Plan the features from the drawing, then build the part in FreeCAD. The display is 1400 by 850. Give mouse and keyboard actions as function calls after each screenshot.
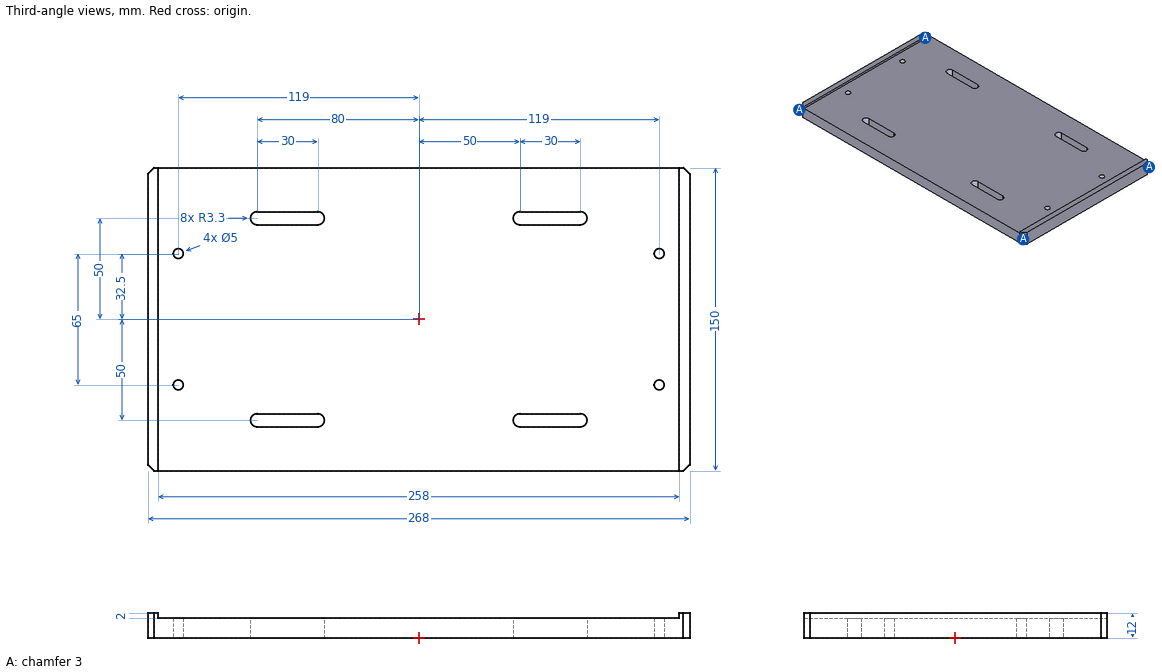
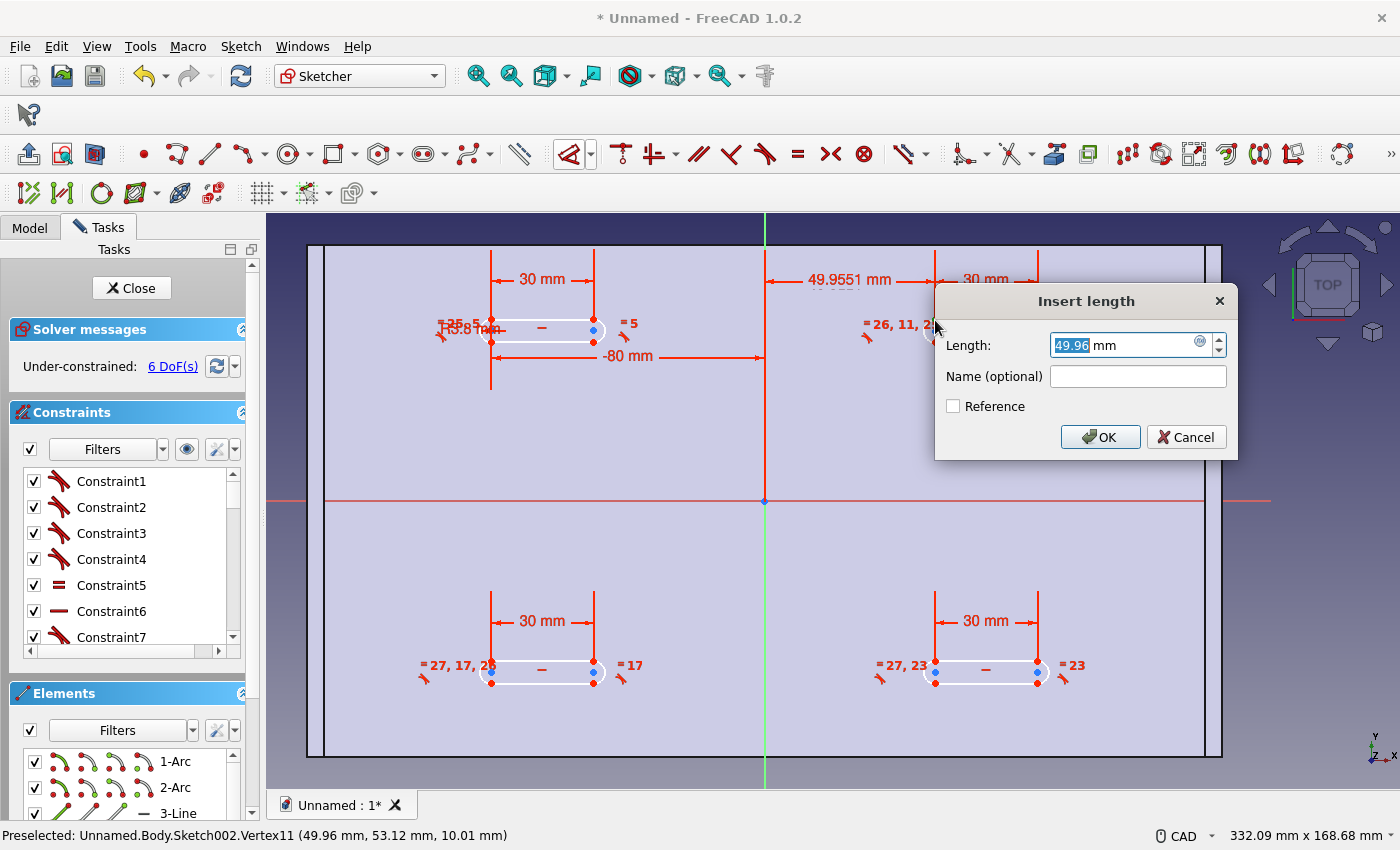
text(50)
key(Return)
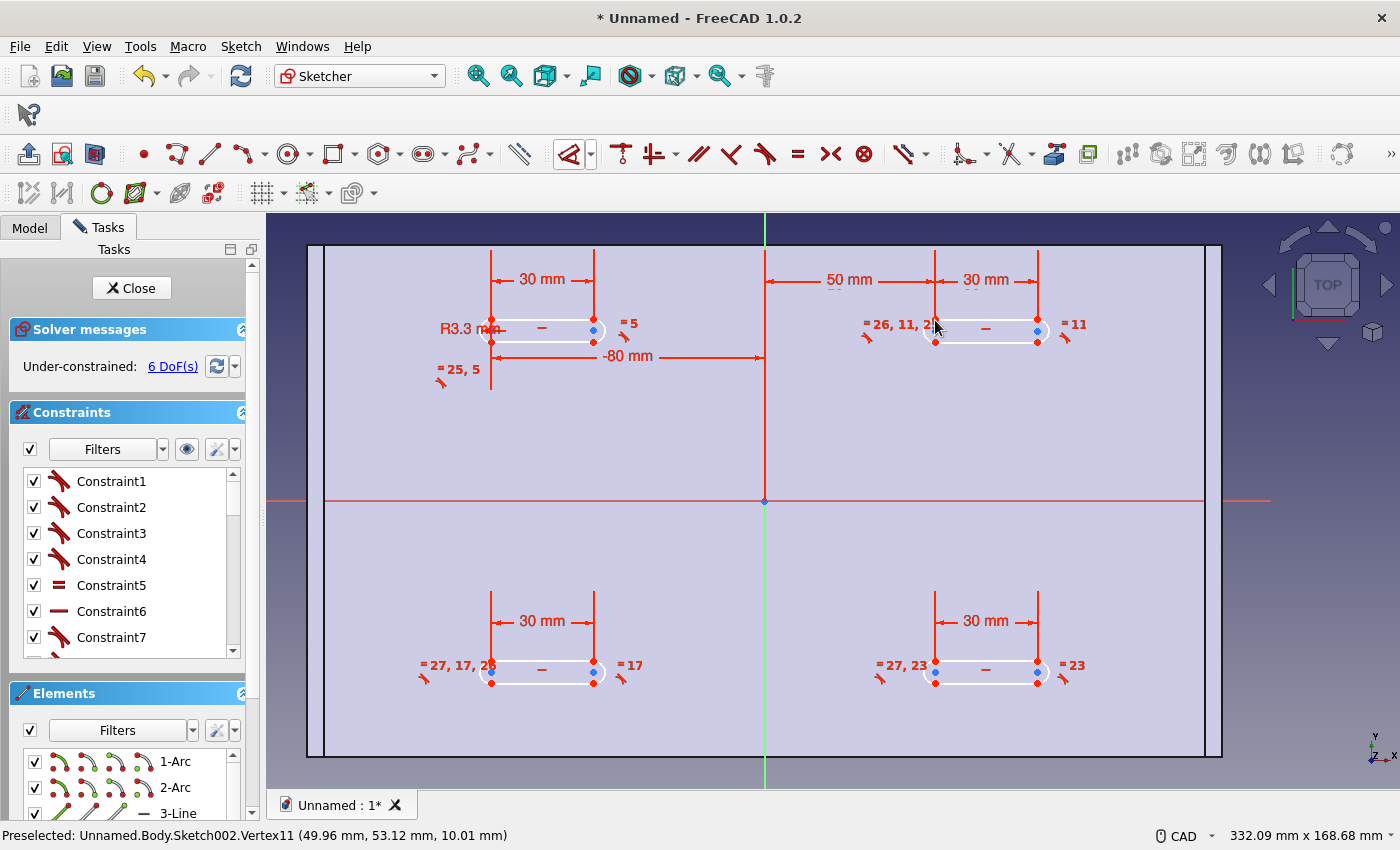
click(491, 661)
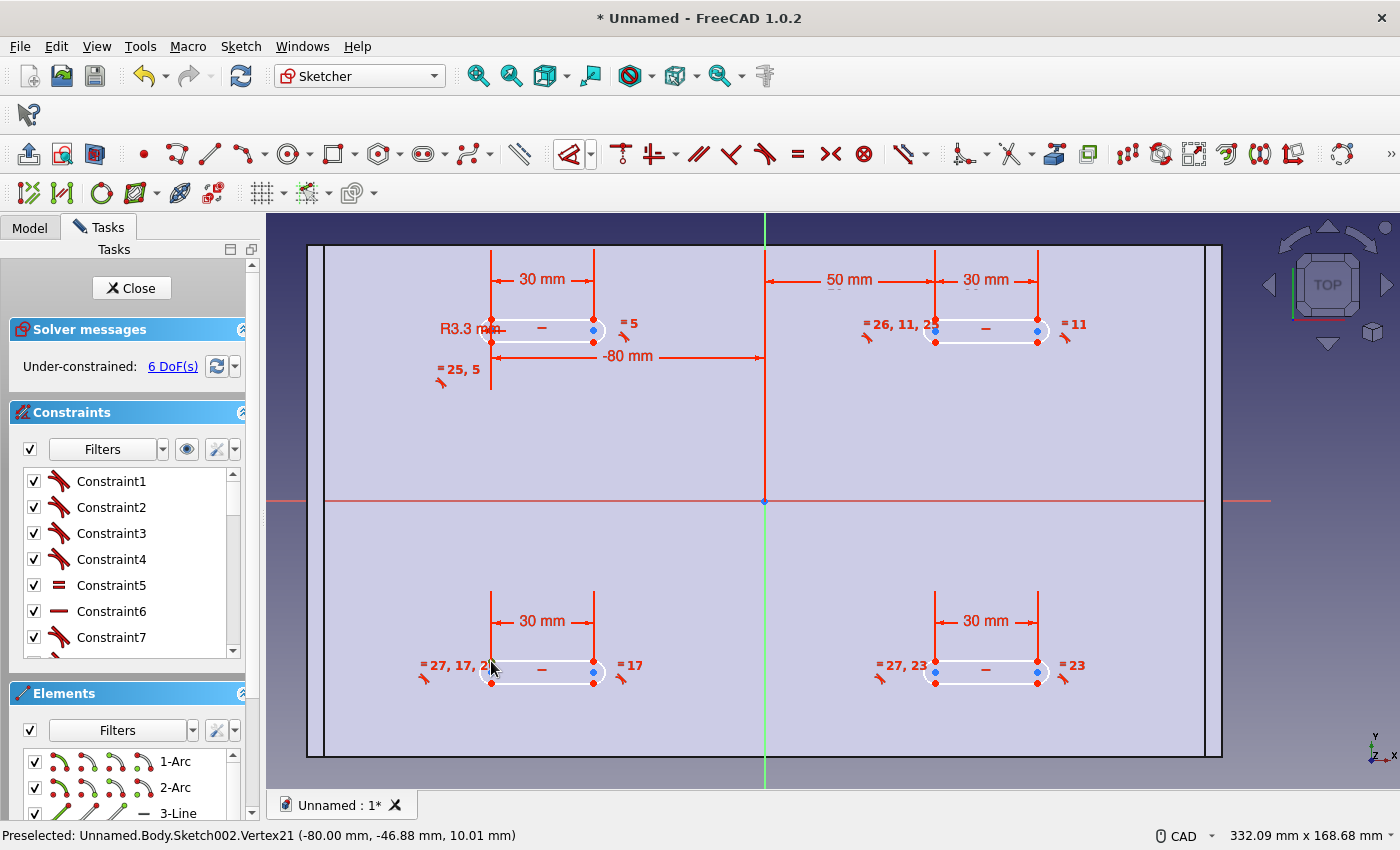
click(590, 154)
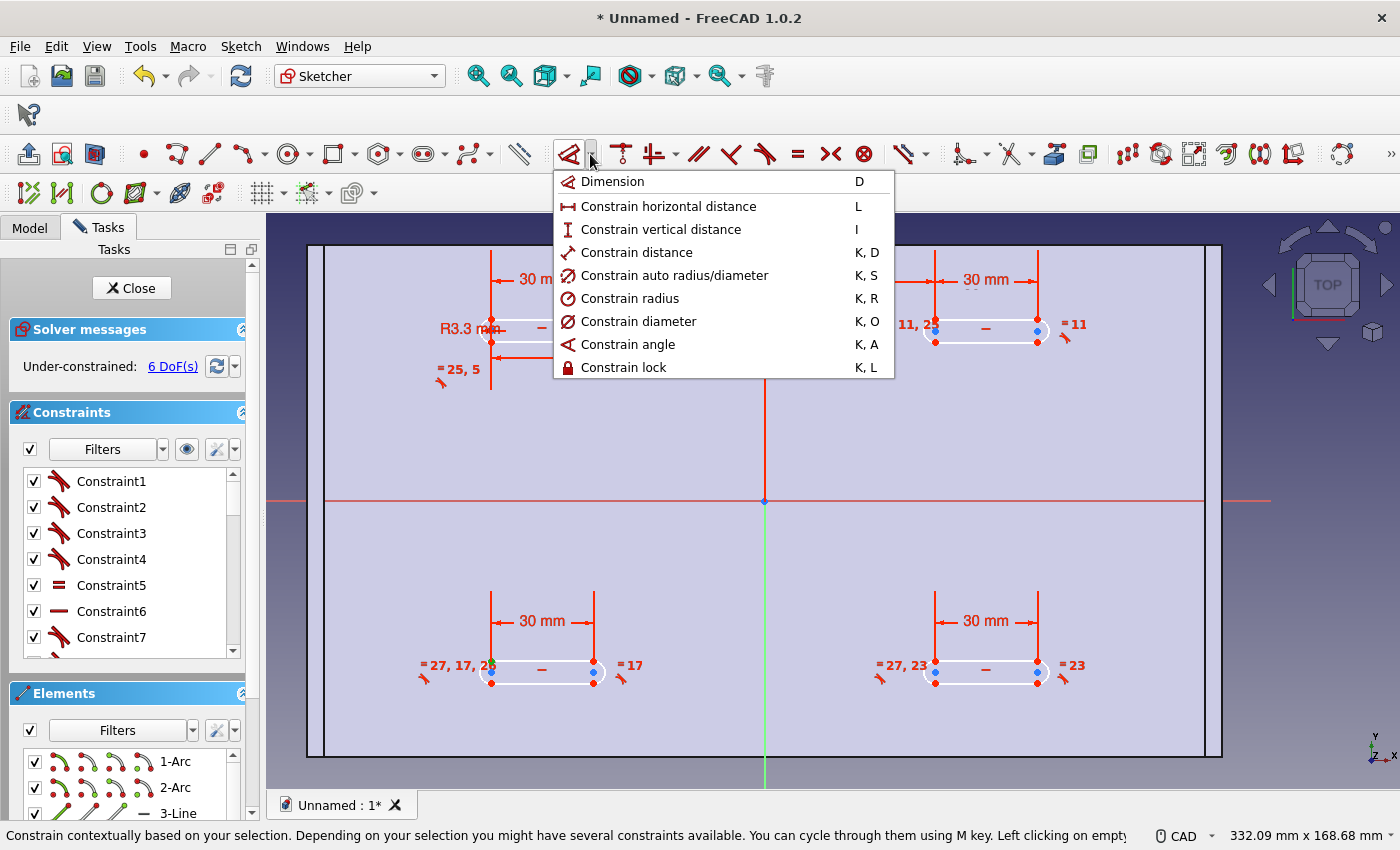
click(724, 206)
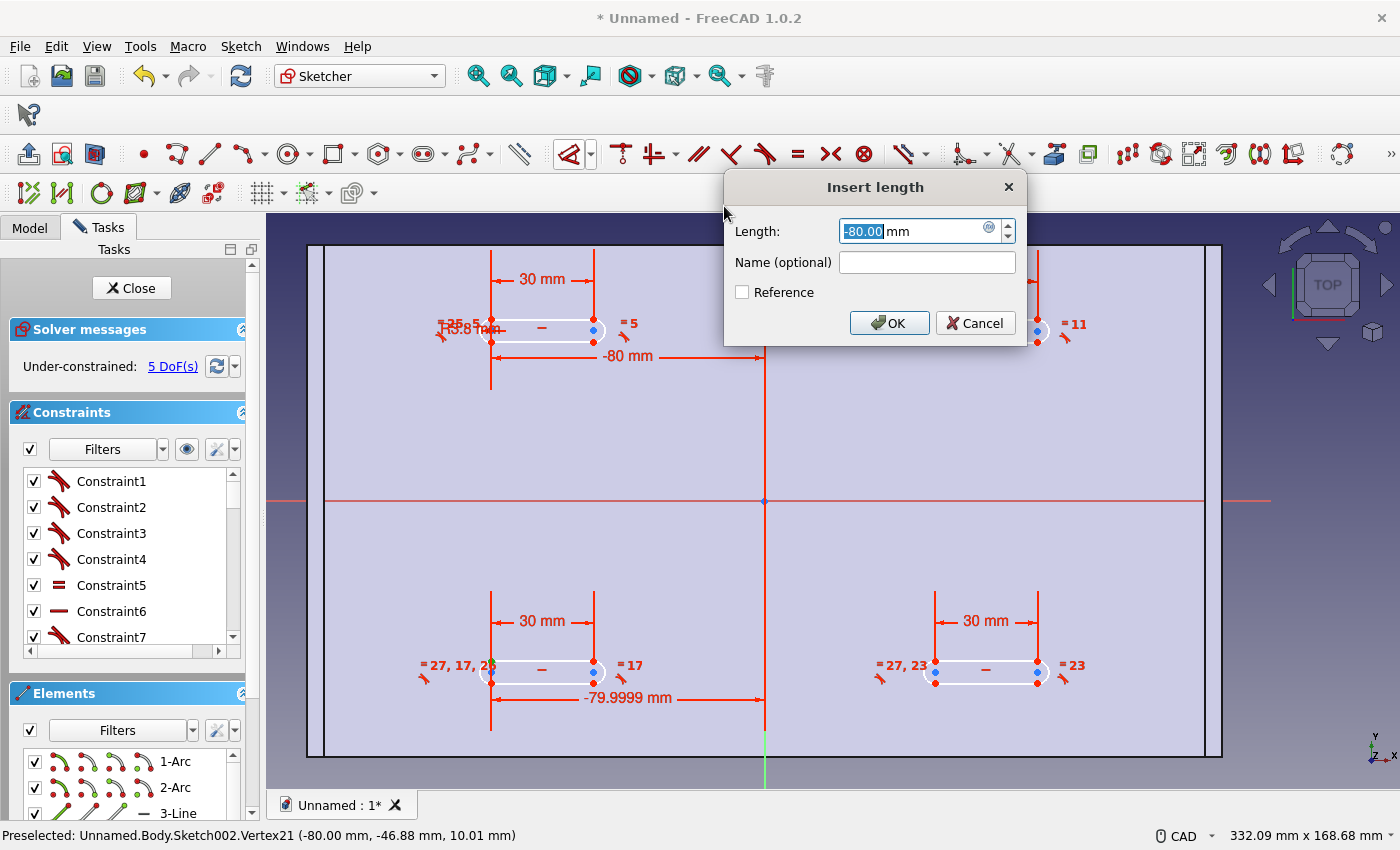
text(-80)
key(Return)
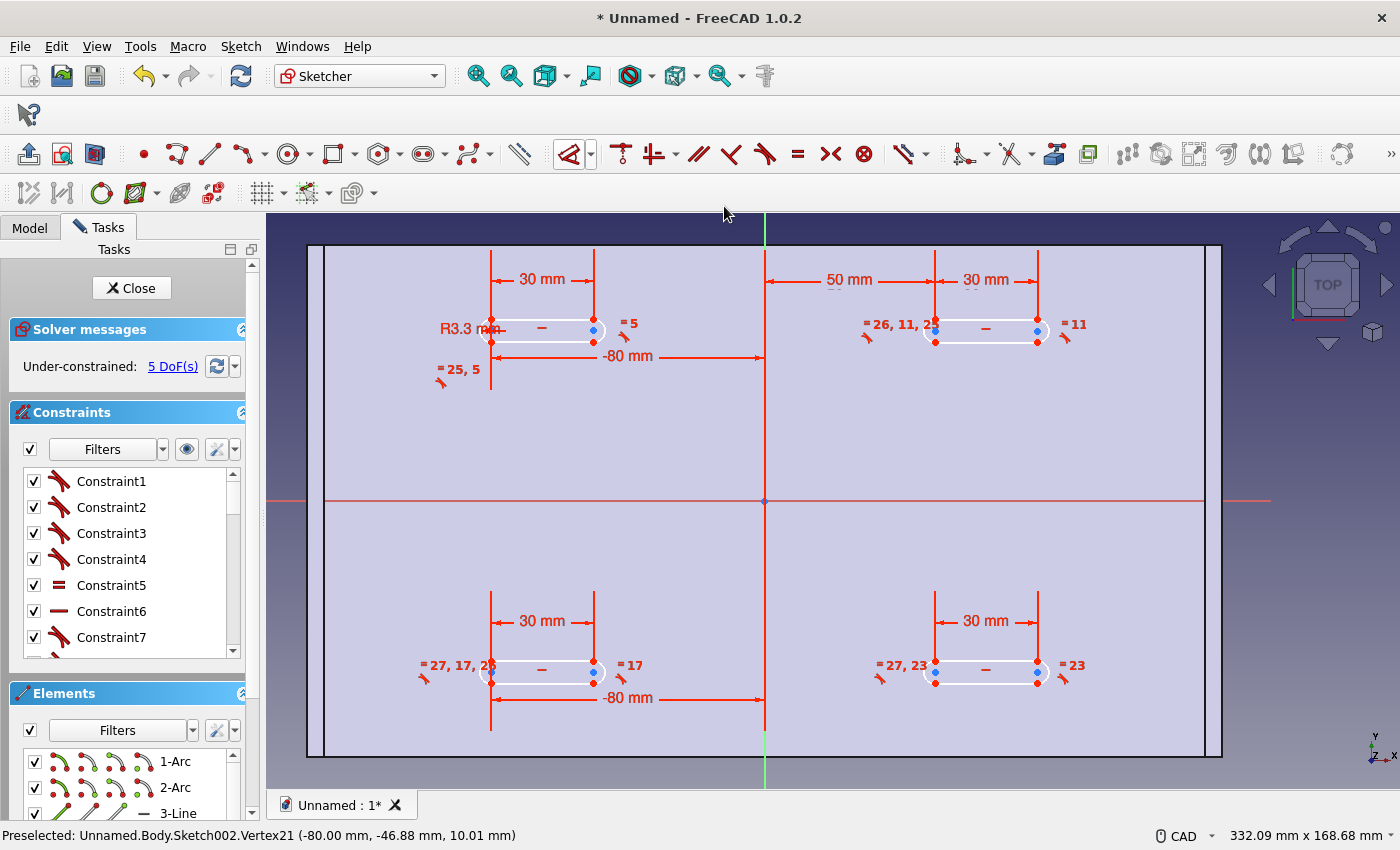
click(935, 661)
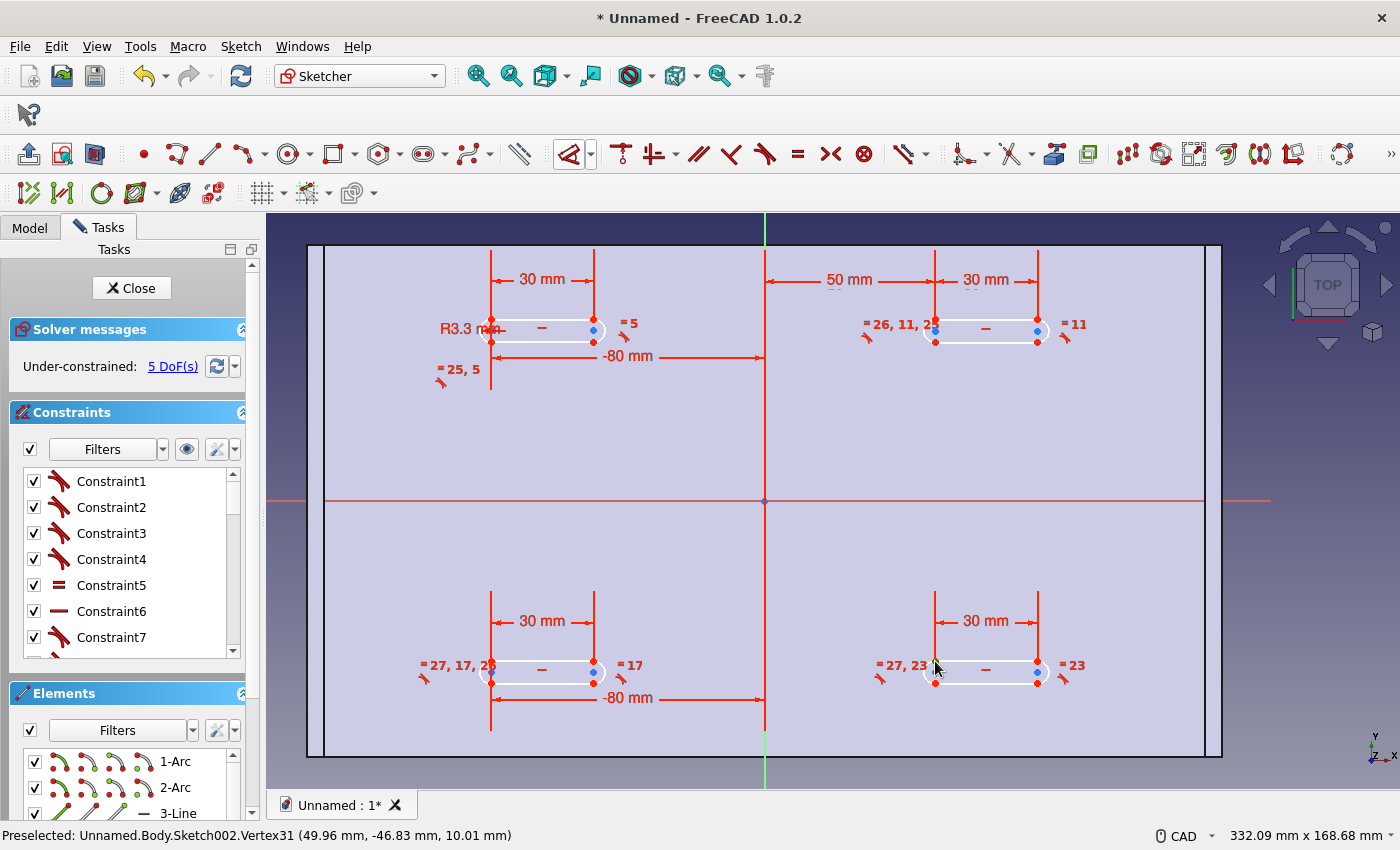
key(l)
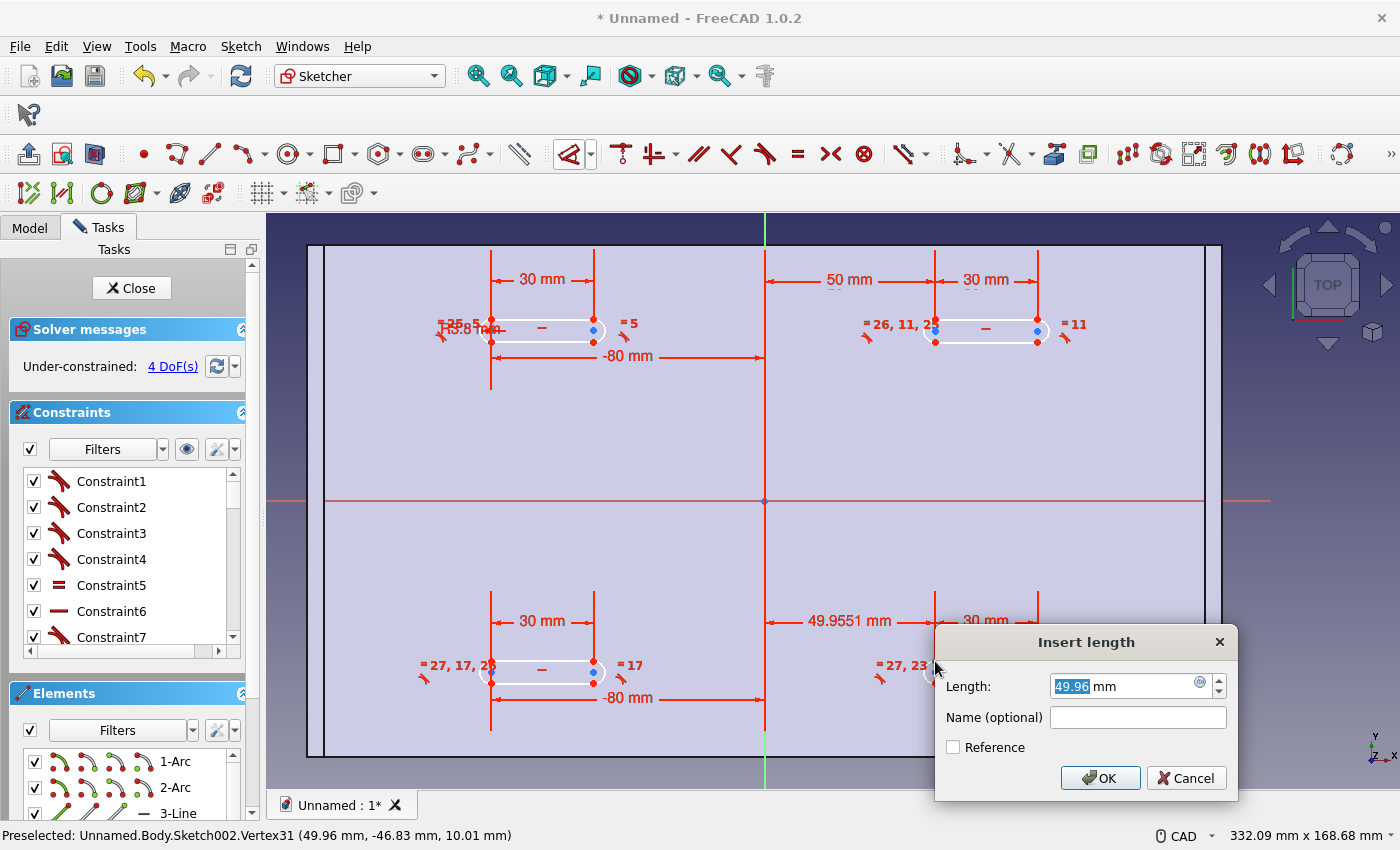
text(50)
key(Return)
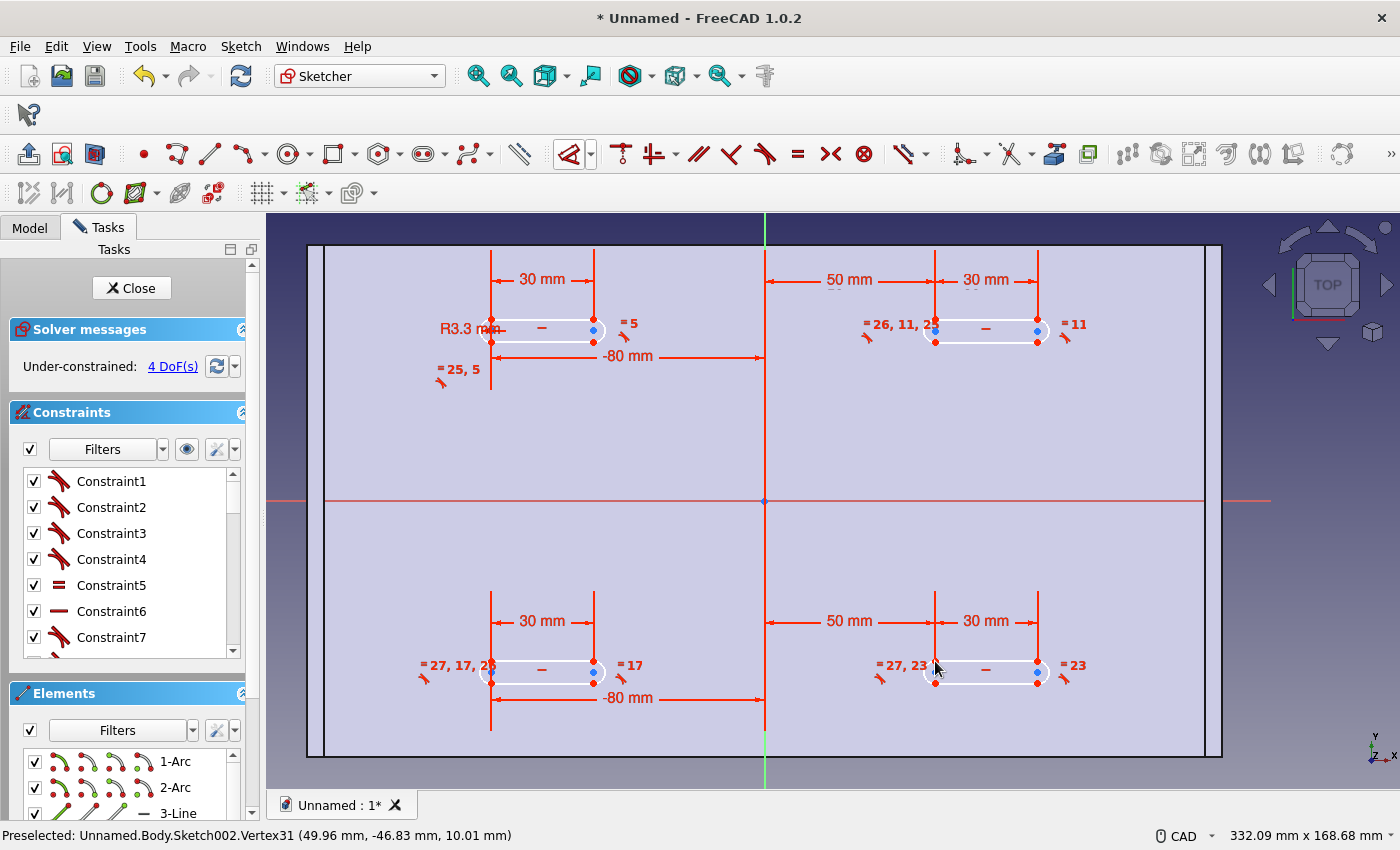
click(491, 331)